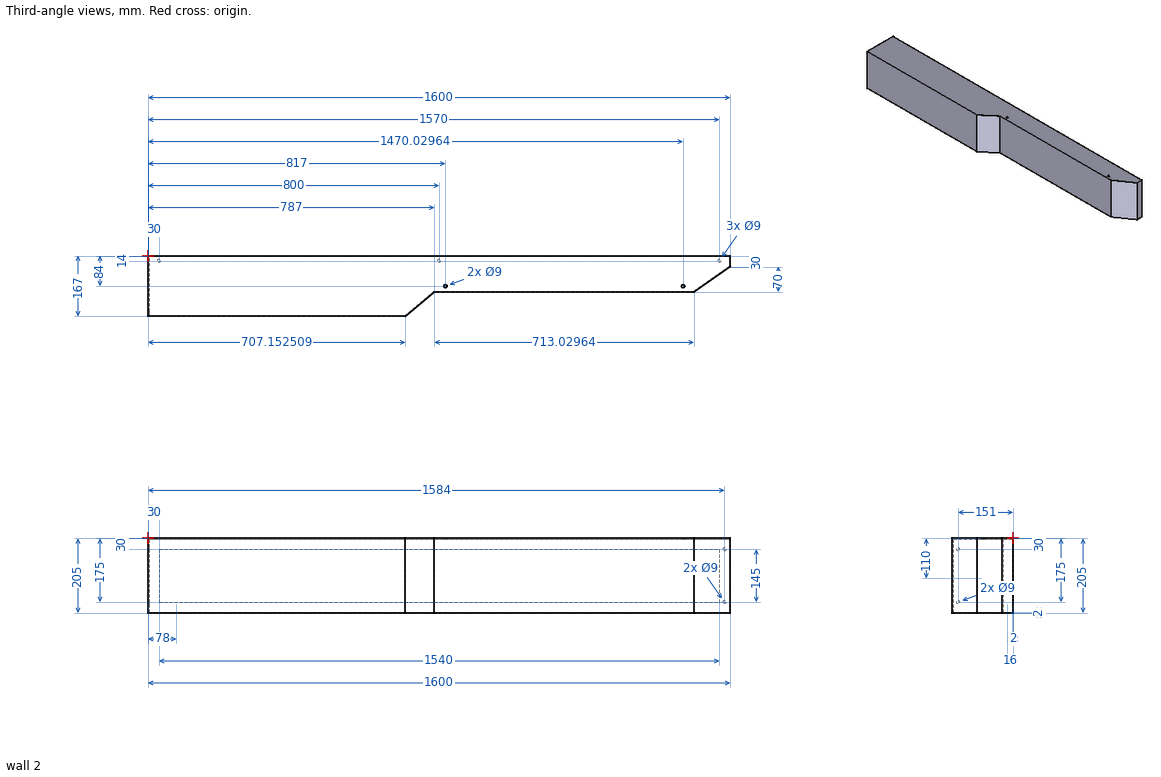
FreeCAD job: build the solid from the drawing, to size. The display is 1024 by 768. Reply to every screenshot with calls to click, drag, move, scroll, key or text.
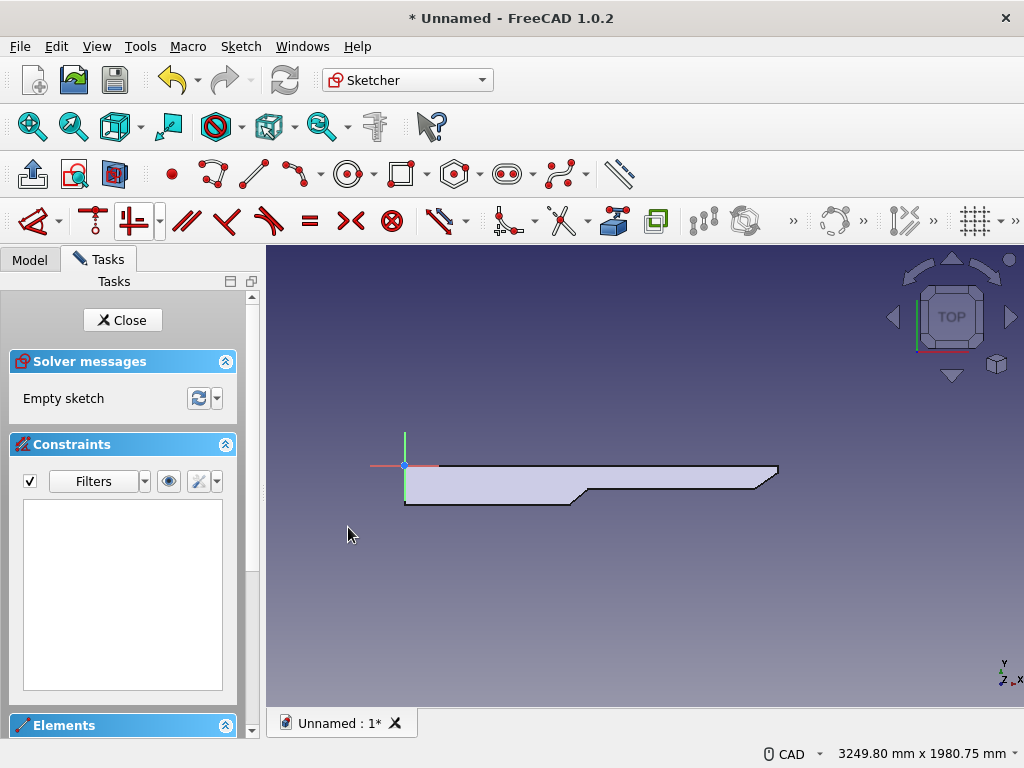
click(348, 174)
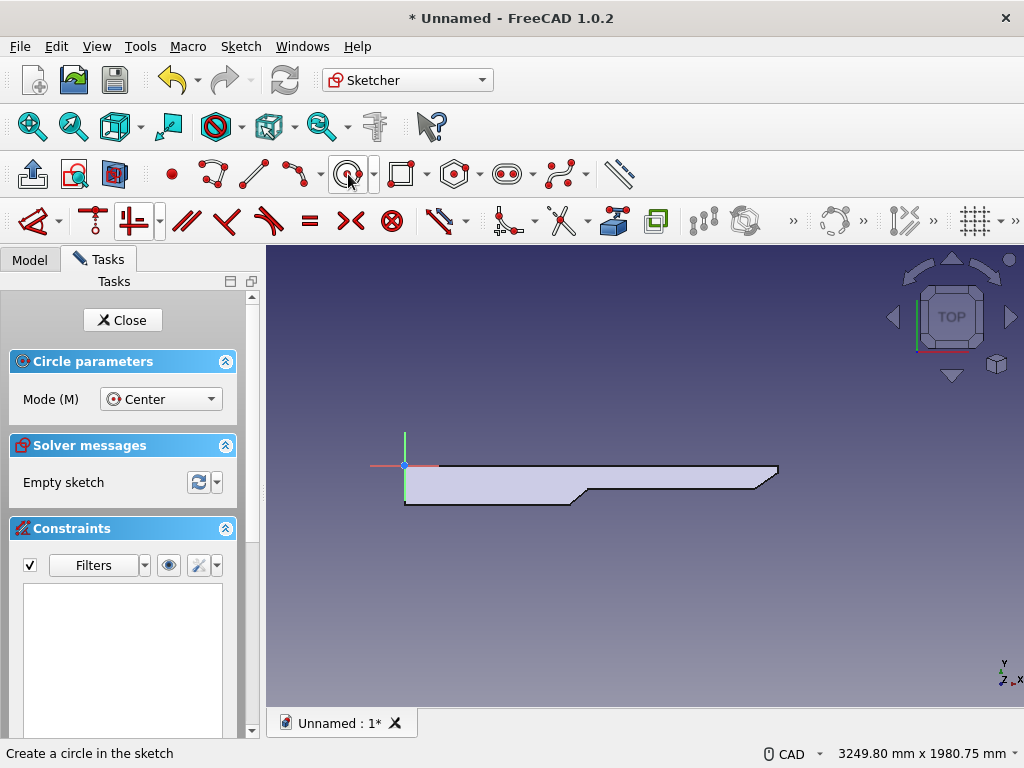
scroll(595, 485, up, 16)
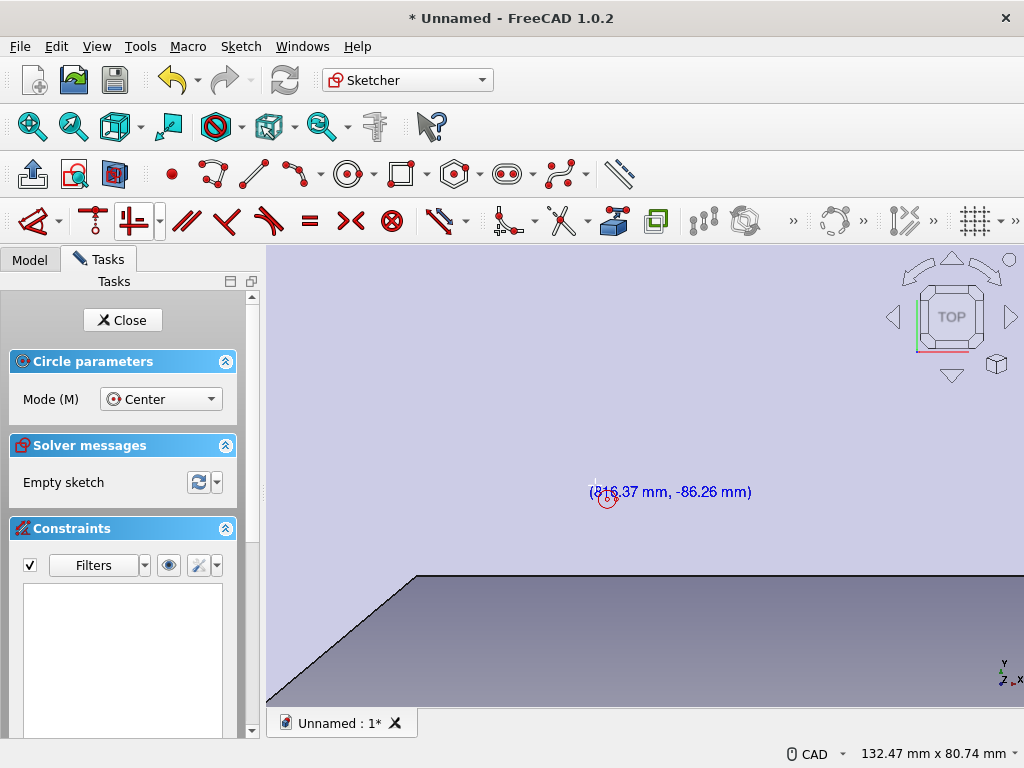
scroll(600, 487, down, 15)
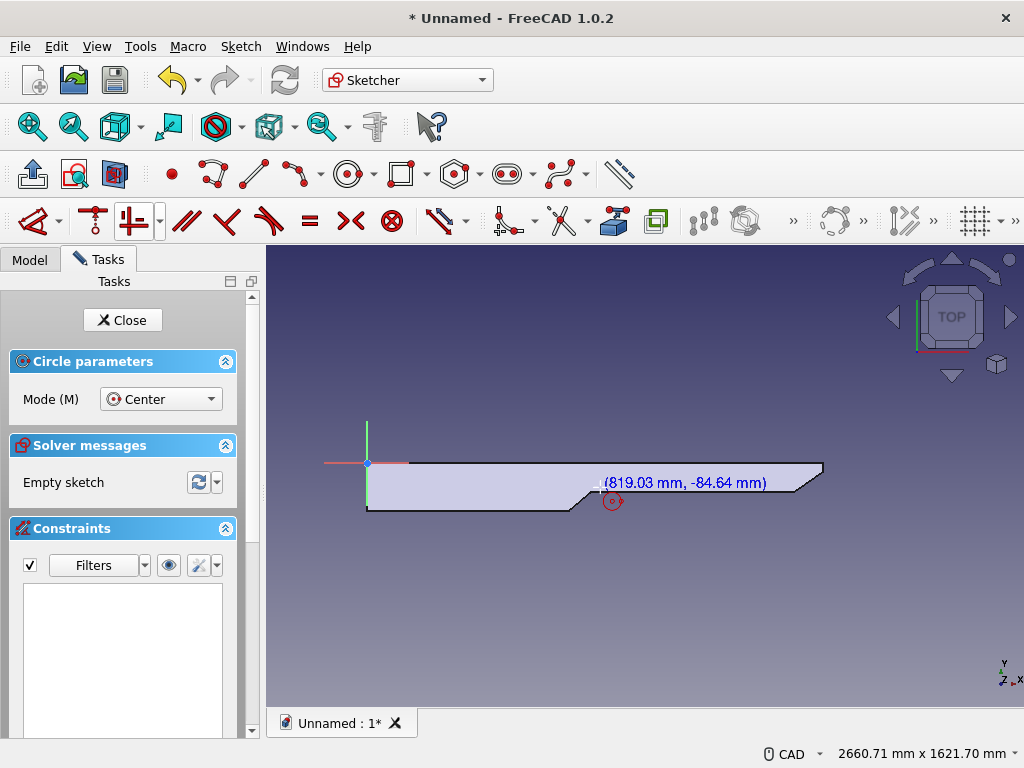
click(600, 487)
move(601, 486)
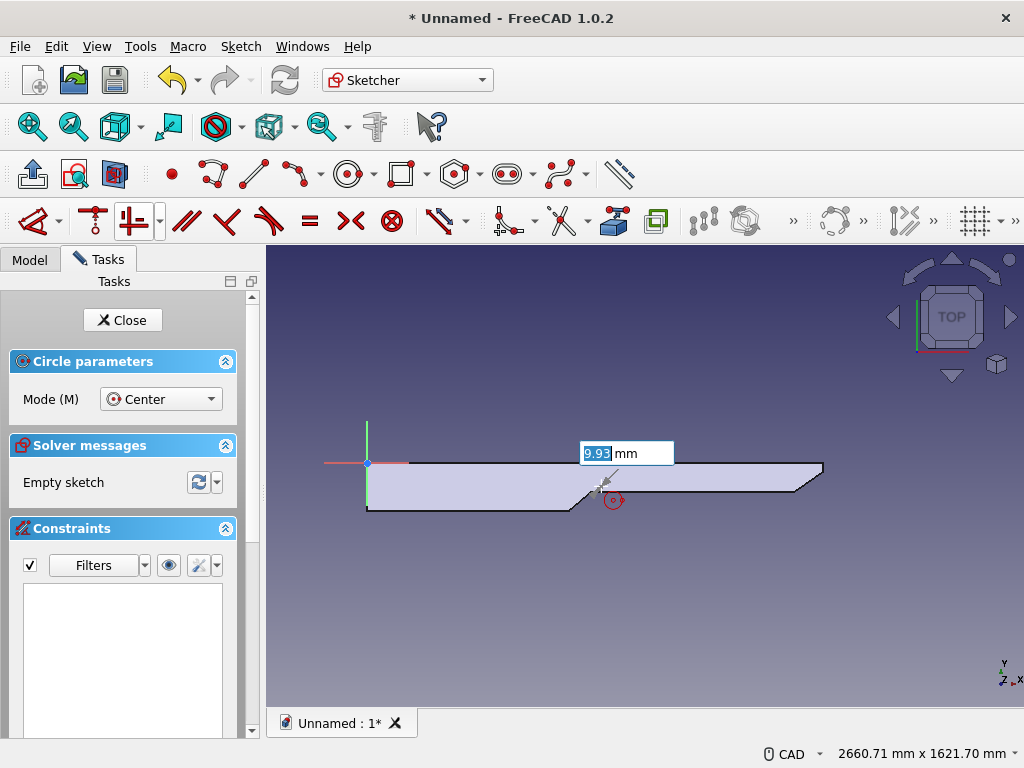
text(9)
key(Return)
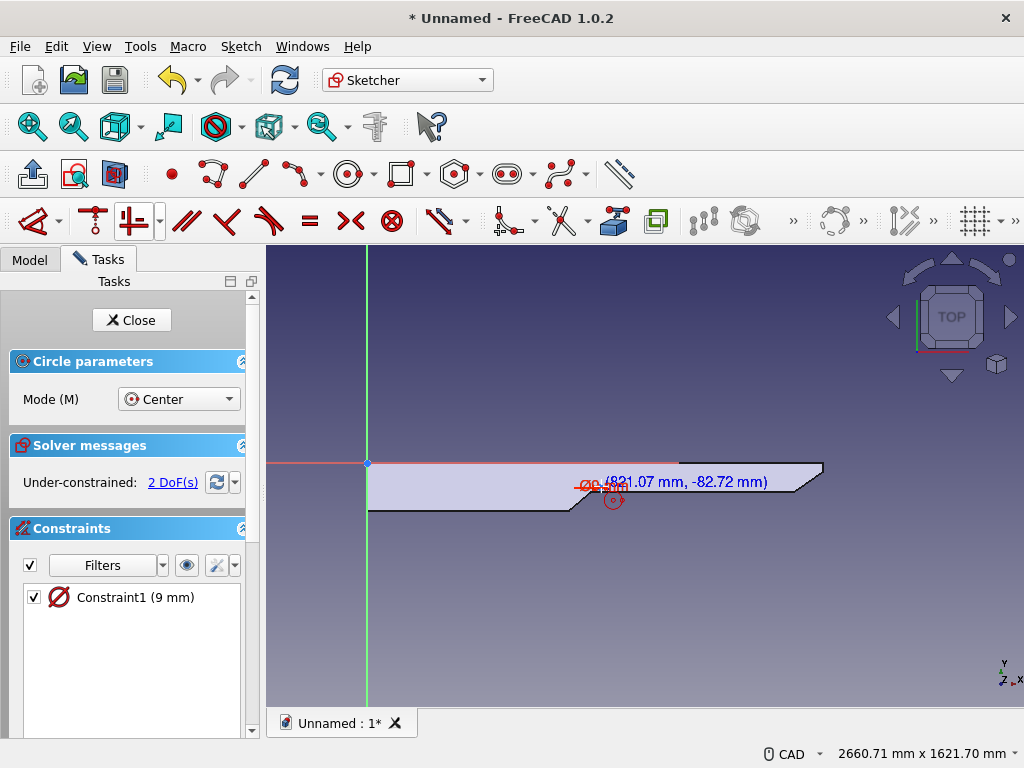
scroll(786, 487, up, 15)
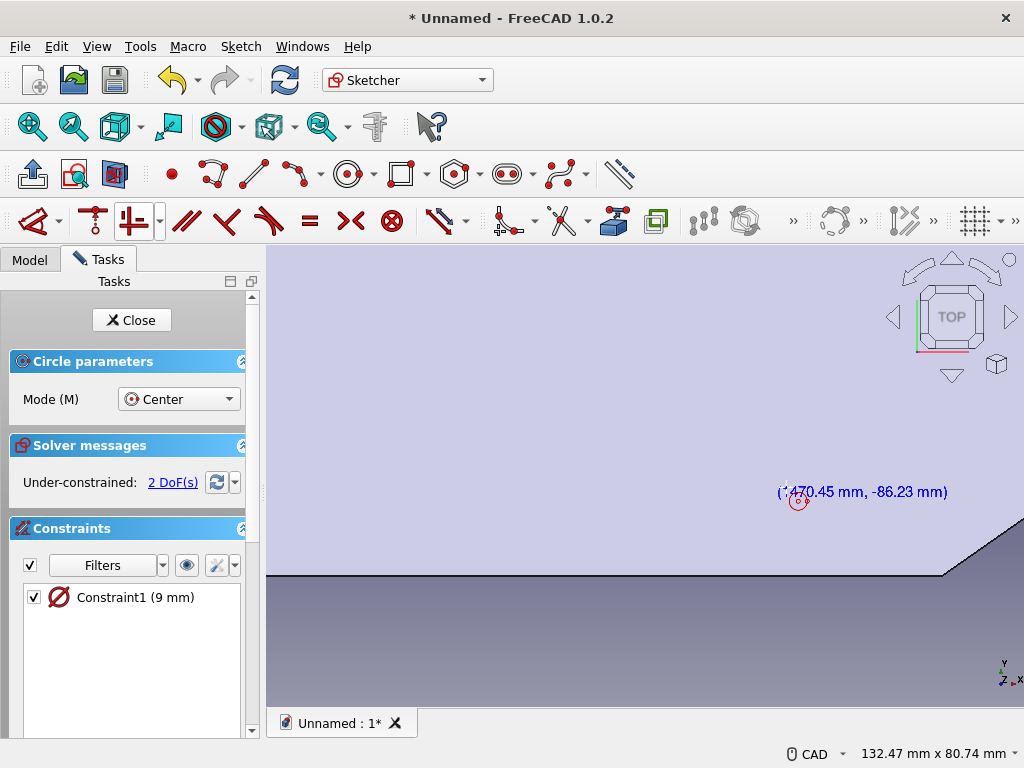
scroll(786, 487, down, 15)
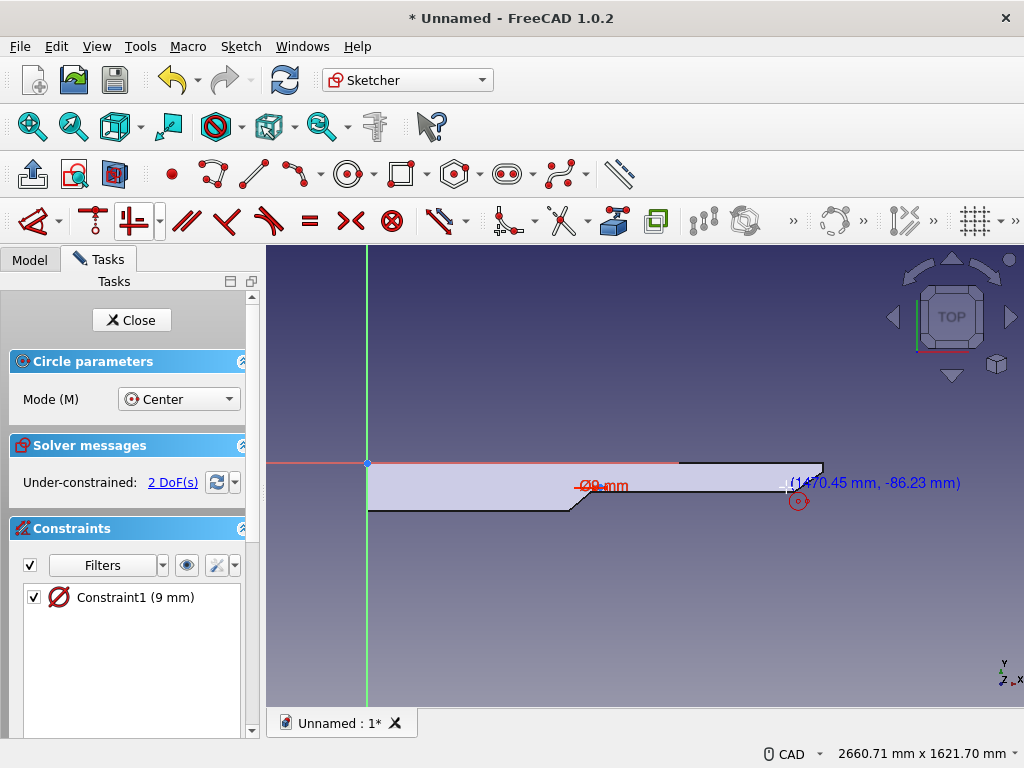
click(786, 487)
move(787, 486)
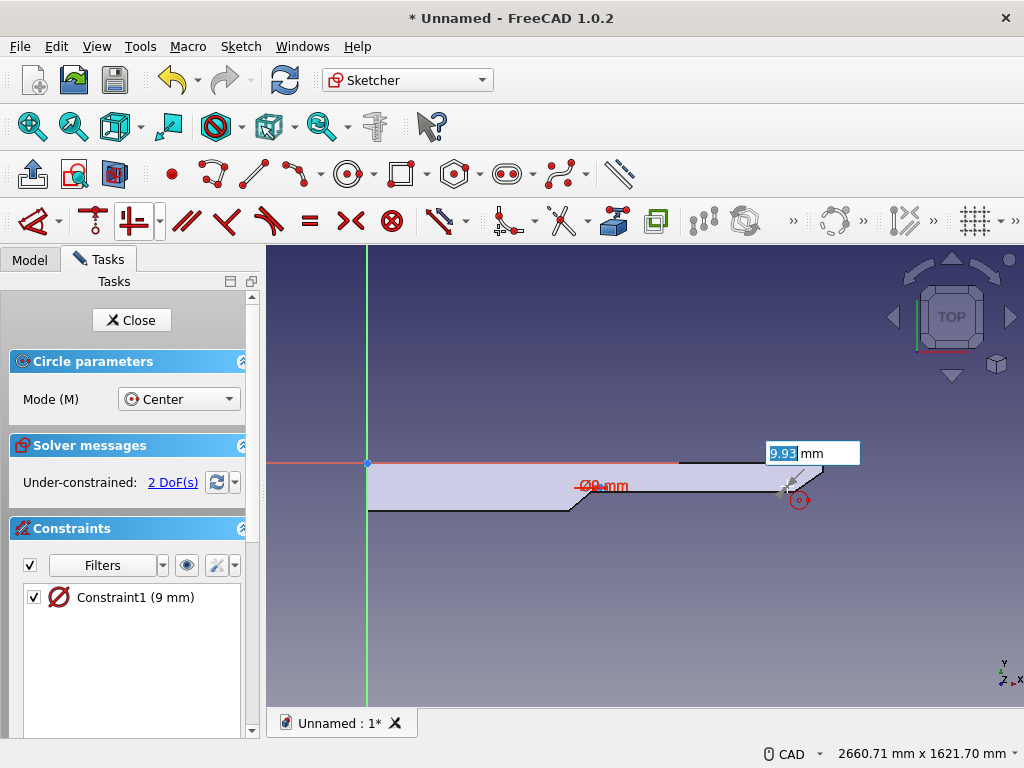
text(9)
key(Return)
key(Escape)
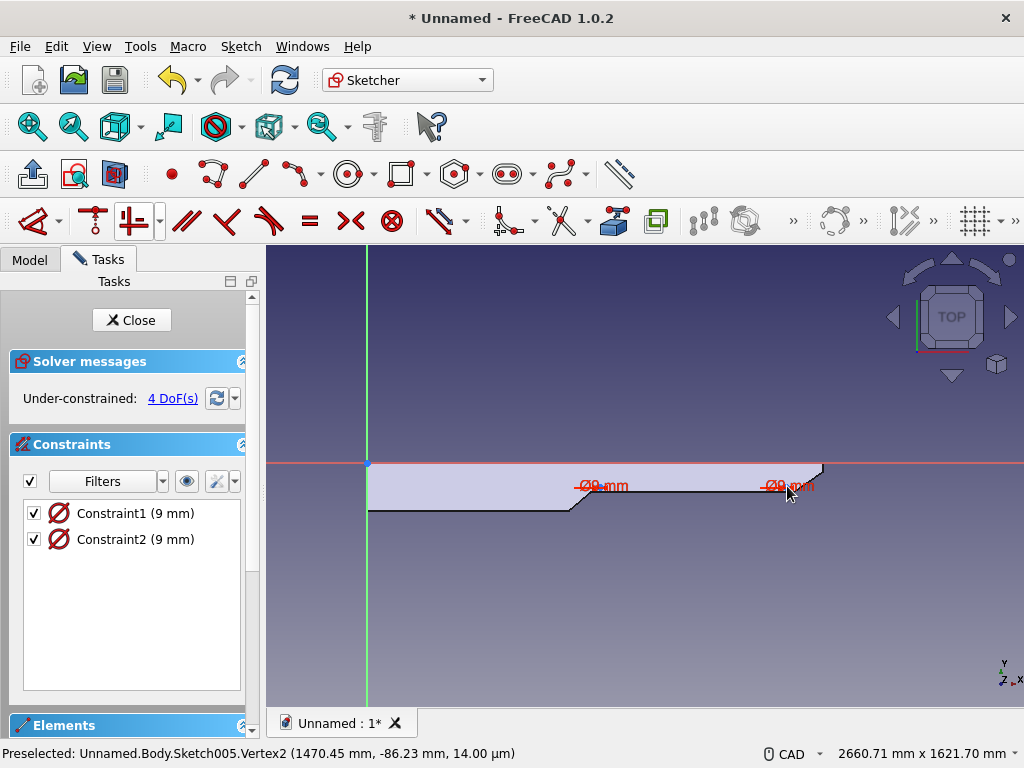
key(d)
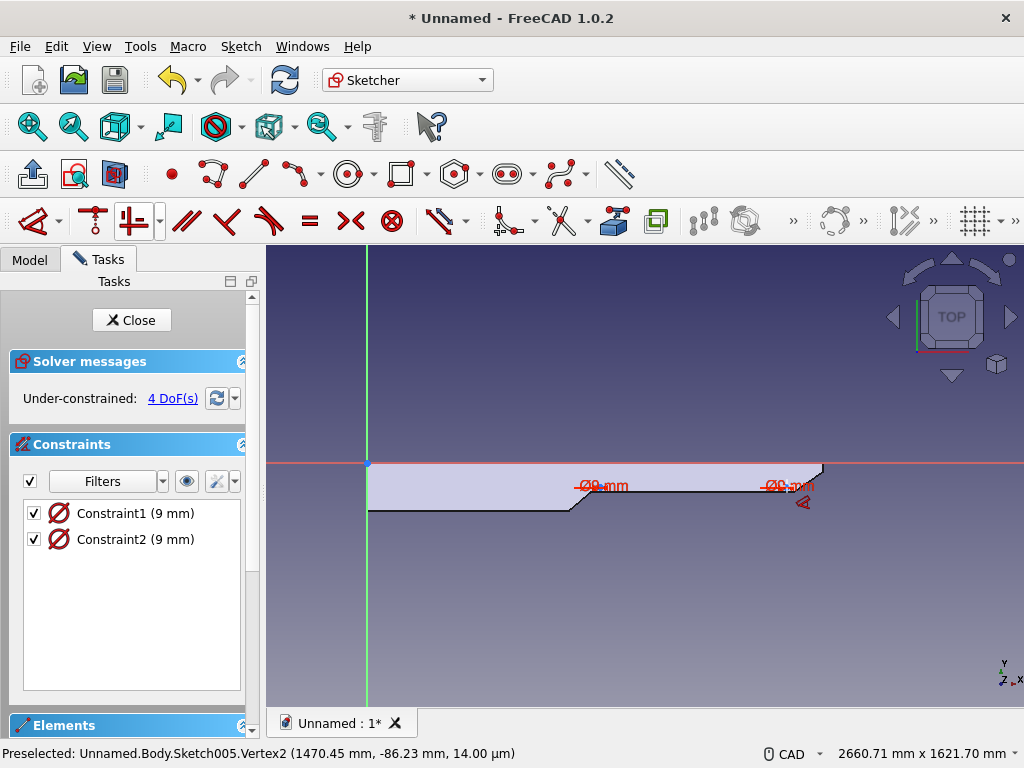
scroll(600, 488, up, 3)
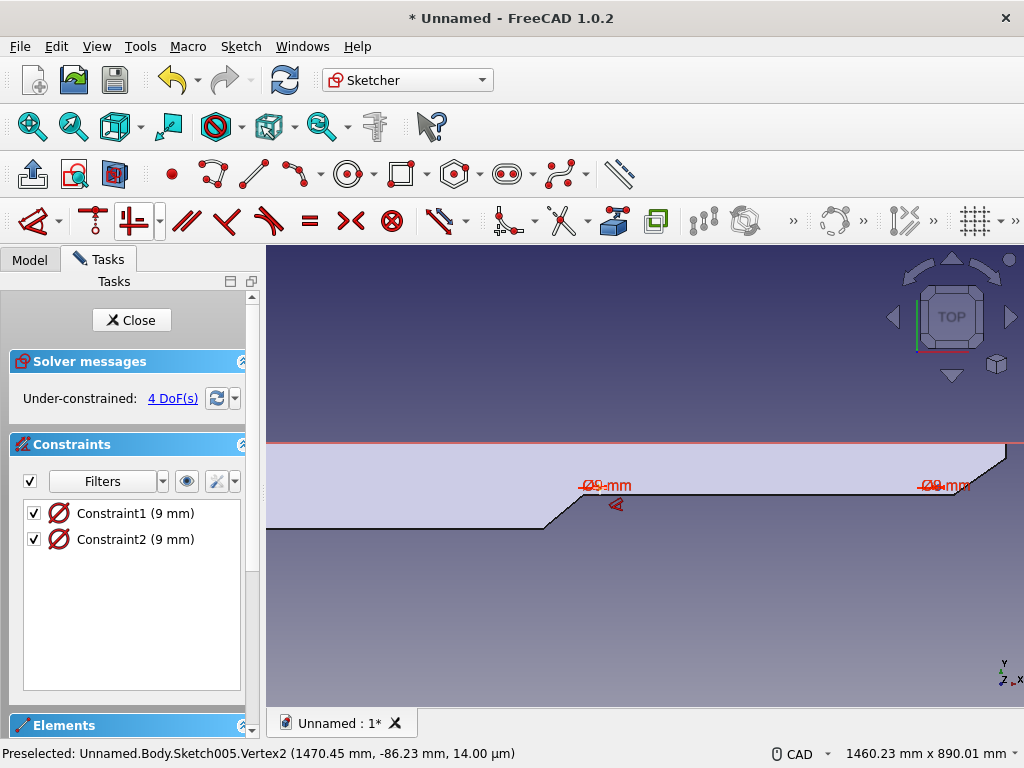
click(600, 488)
click(634, 465)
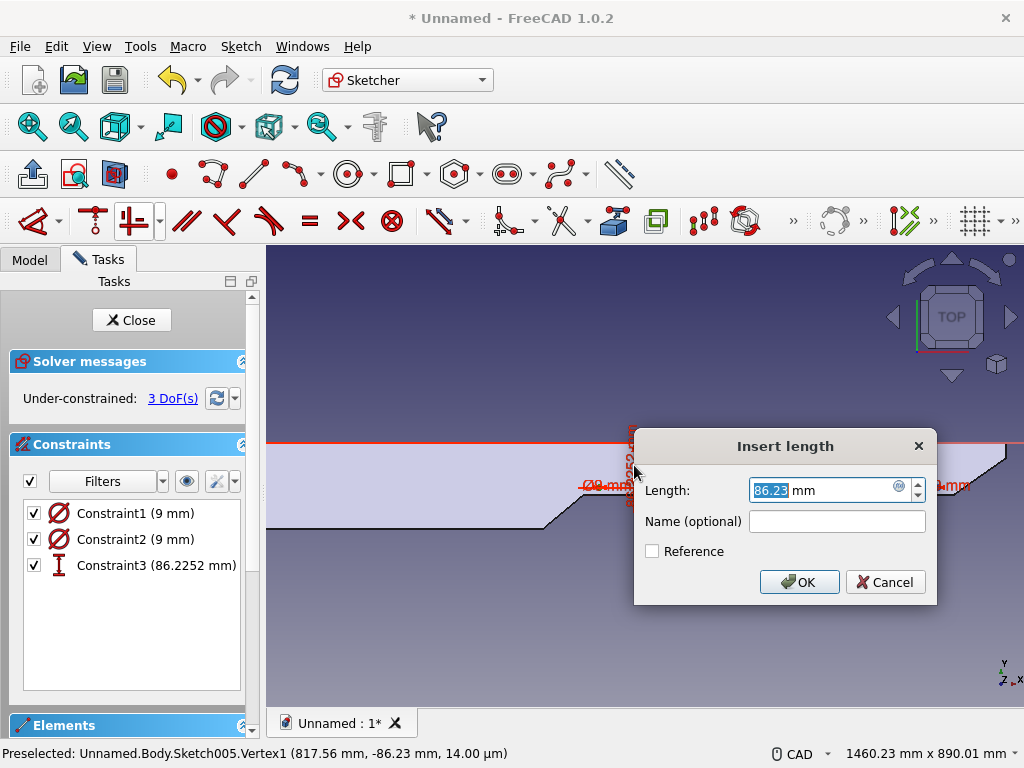
text(84)
key(Return)